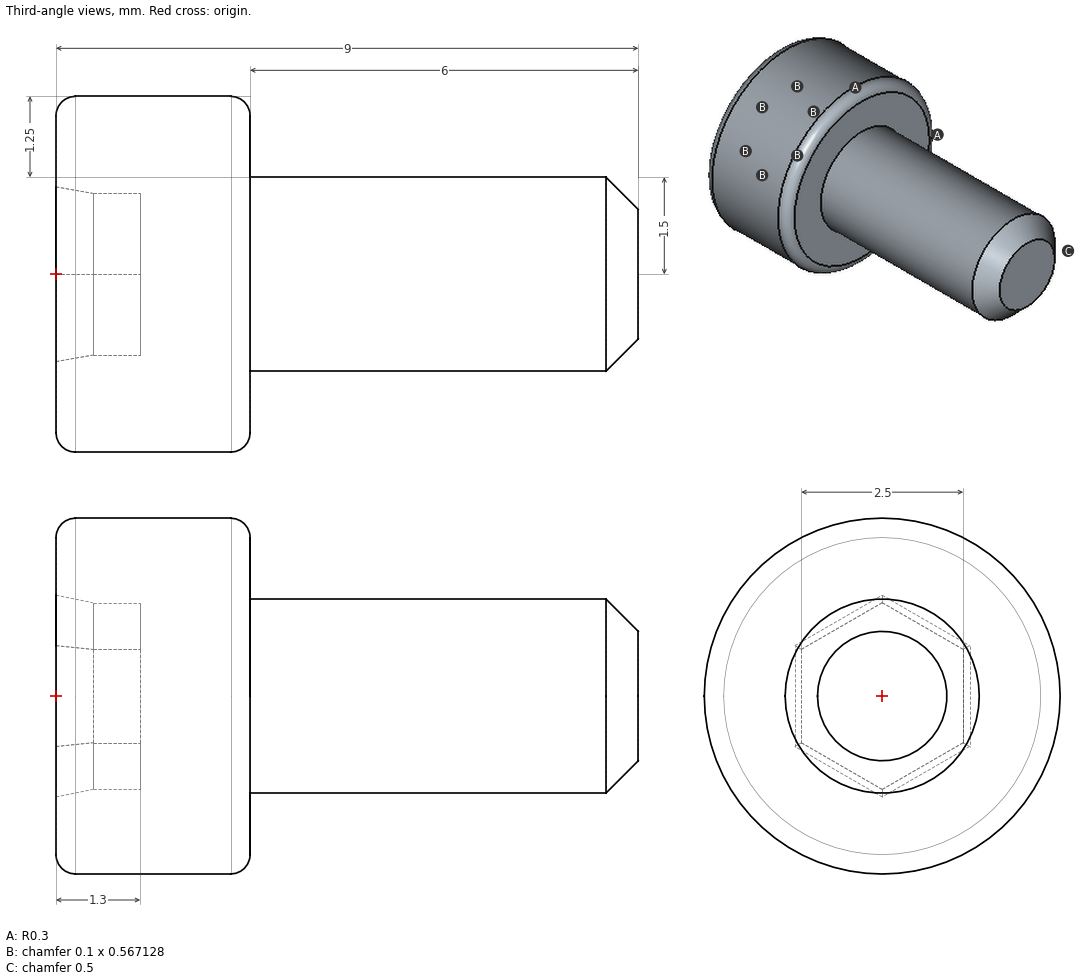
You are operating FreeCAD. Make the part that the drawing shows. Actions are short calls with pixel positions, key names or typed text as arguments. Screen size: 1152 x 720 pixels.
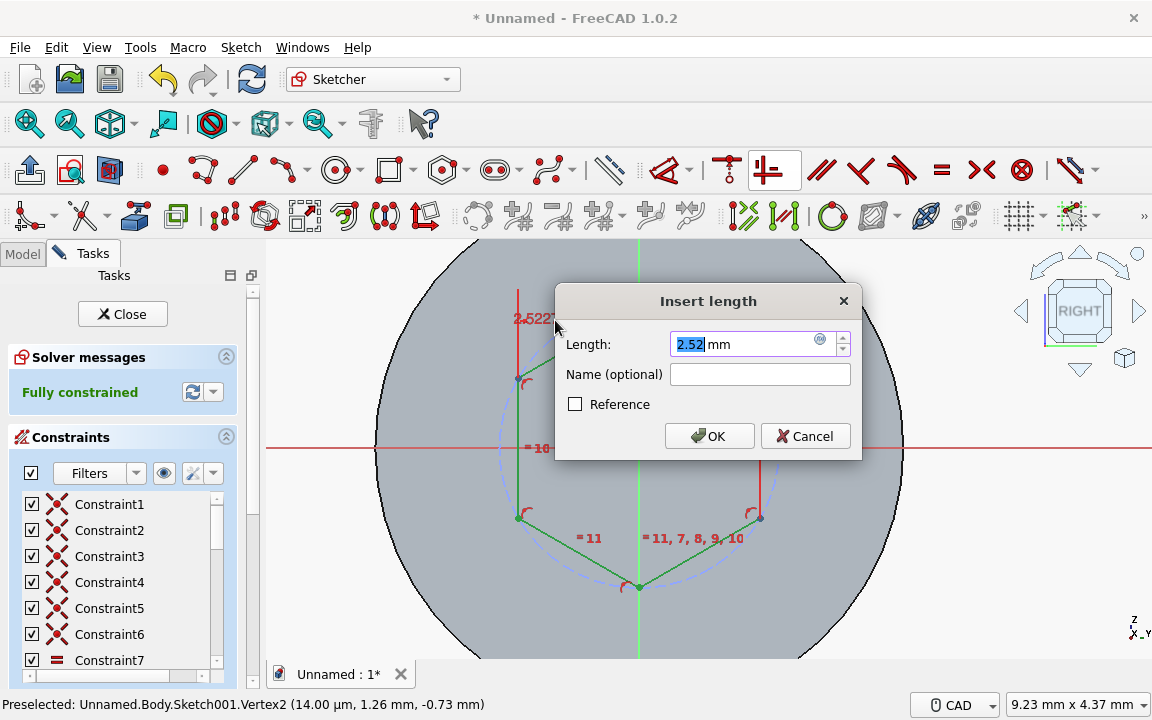
text(2.5)
key(Return)
key(Escape)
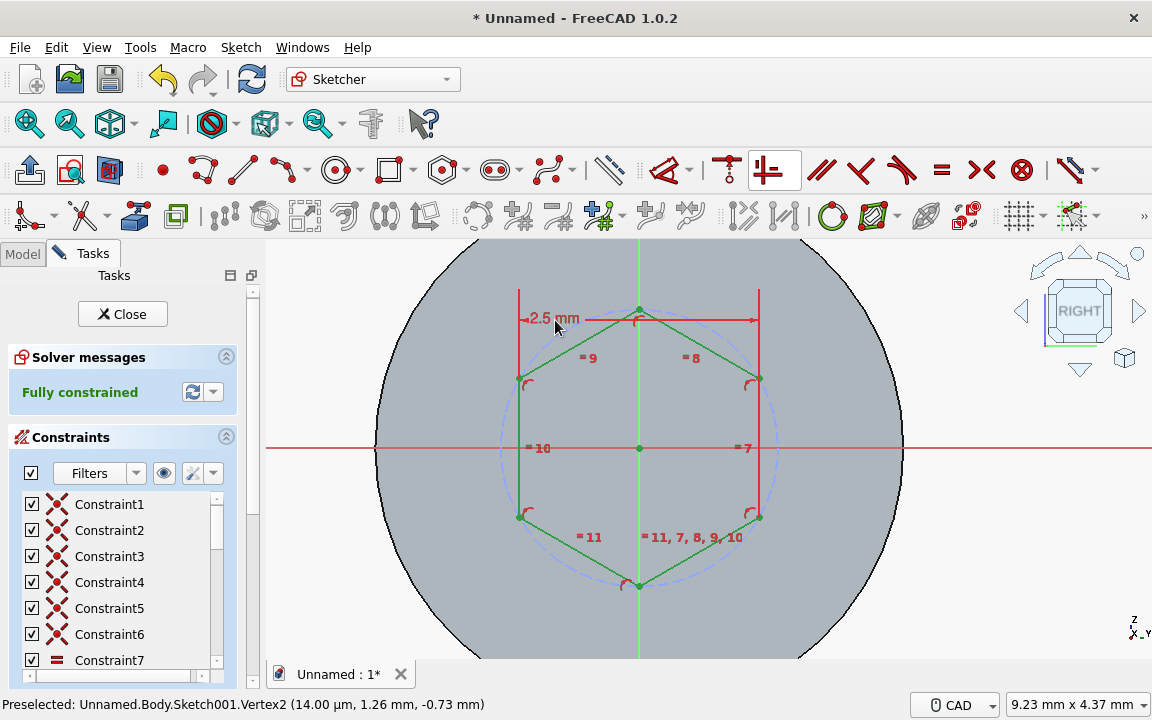
click(123, 314)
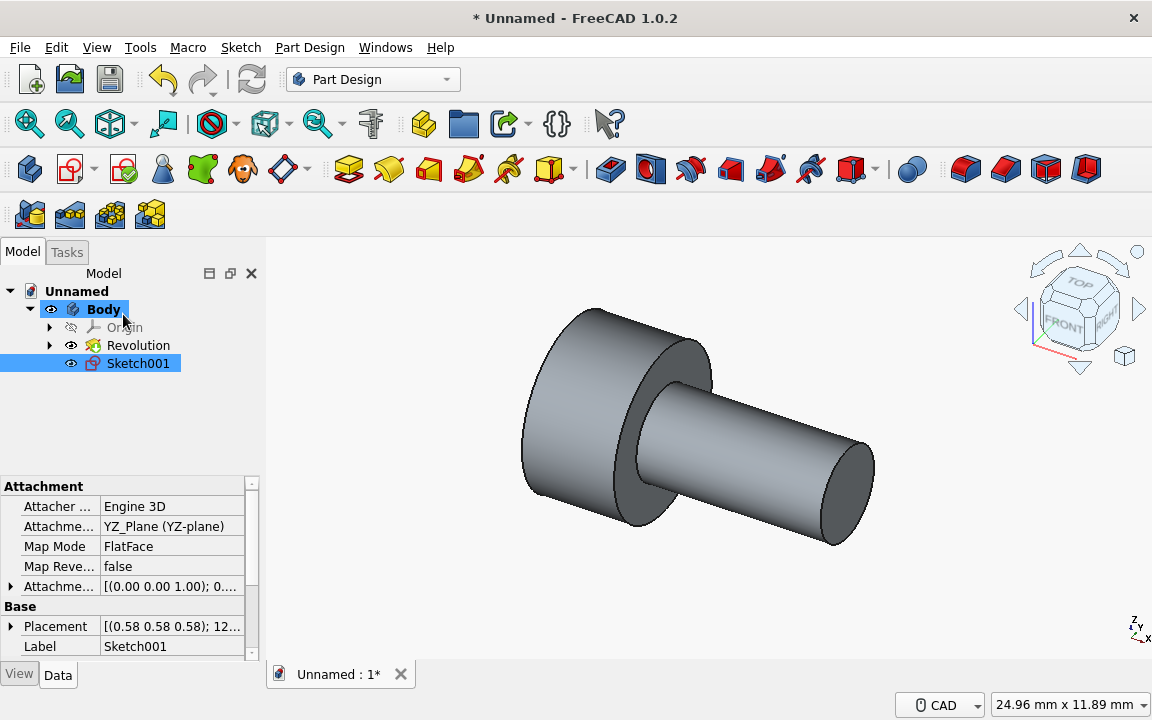
click(612, 170)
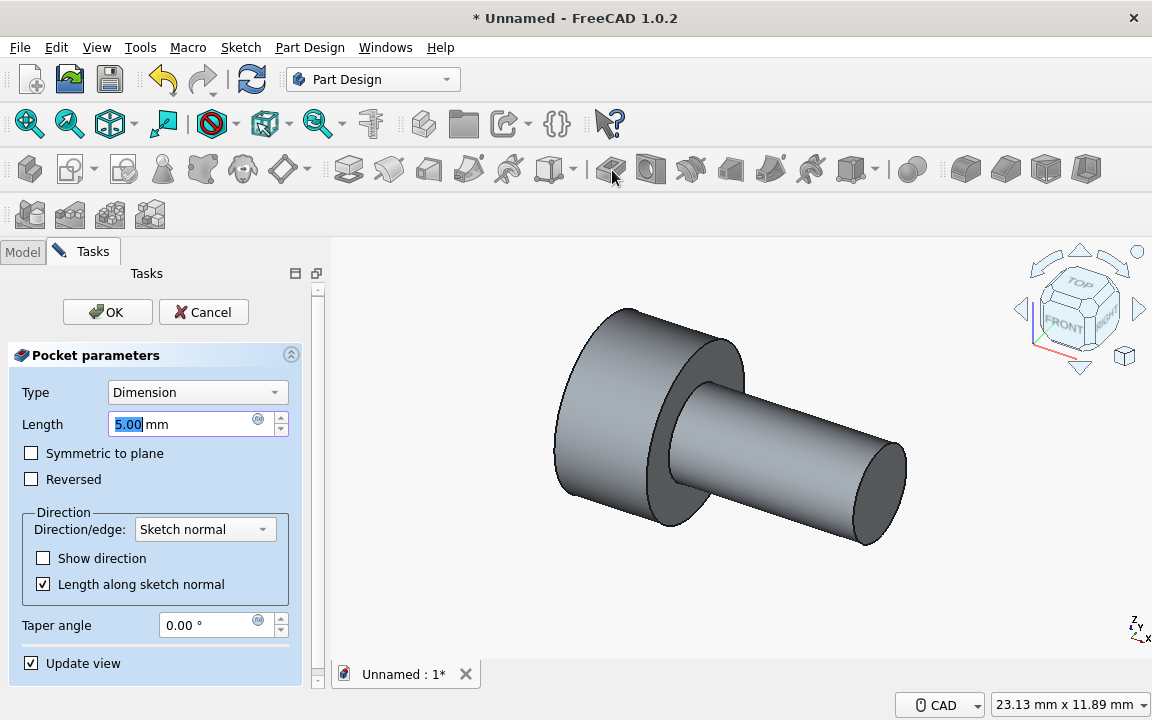
text(1.3)
key(Tab)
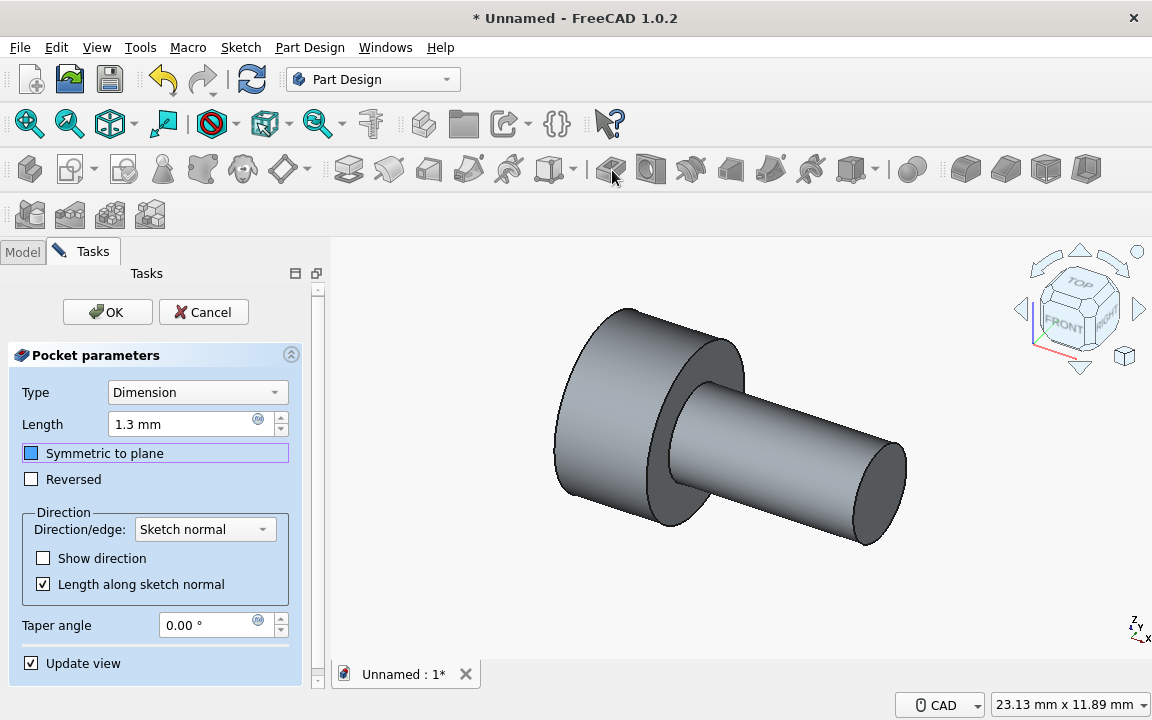
click(30, 479)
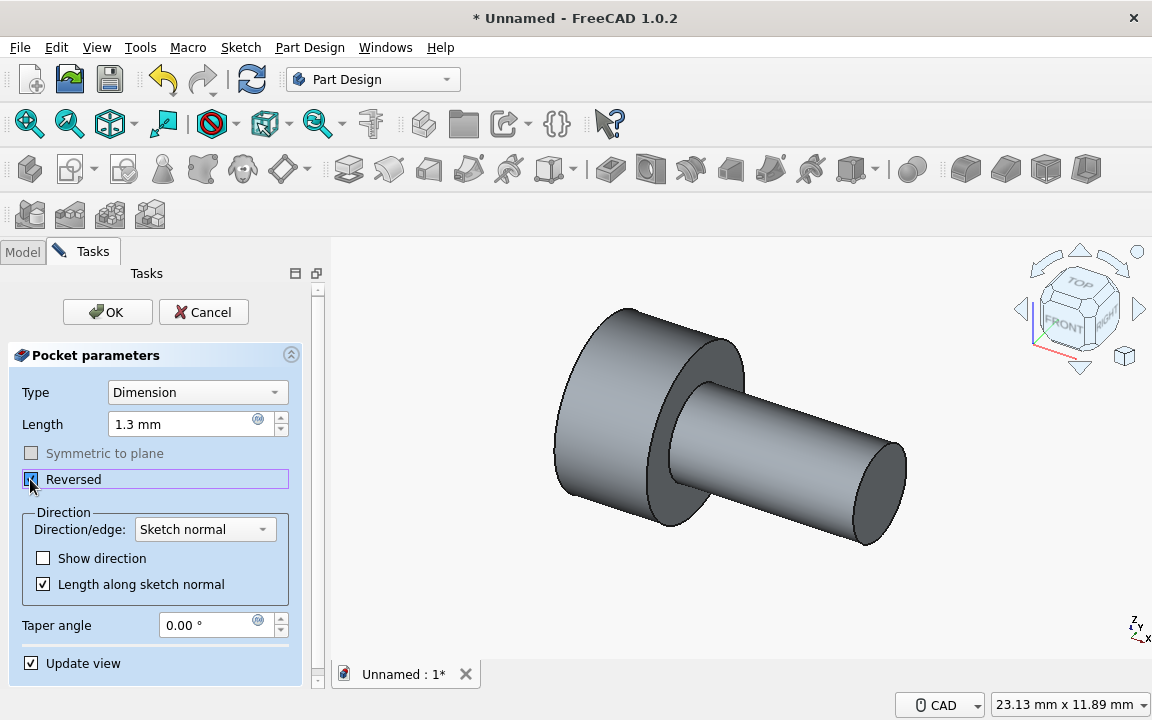
click(108, 312)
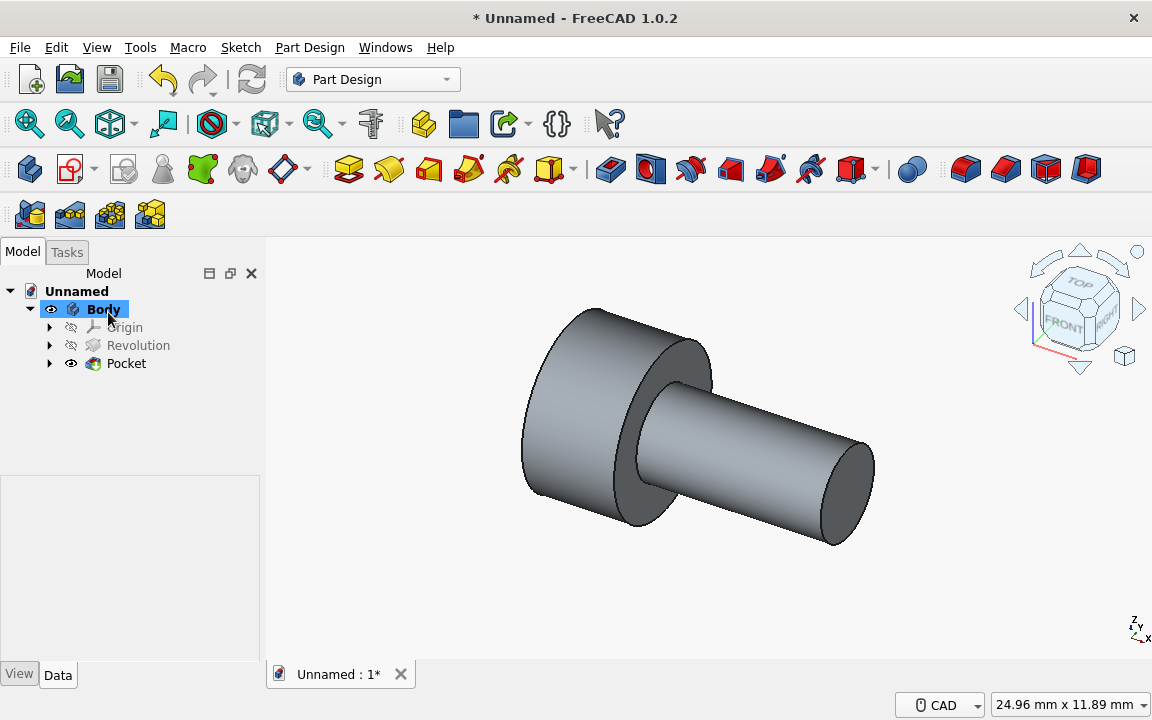
click(614, 480)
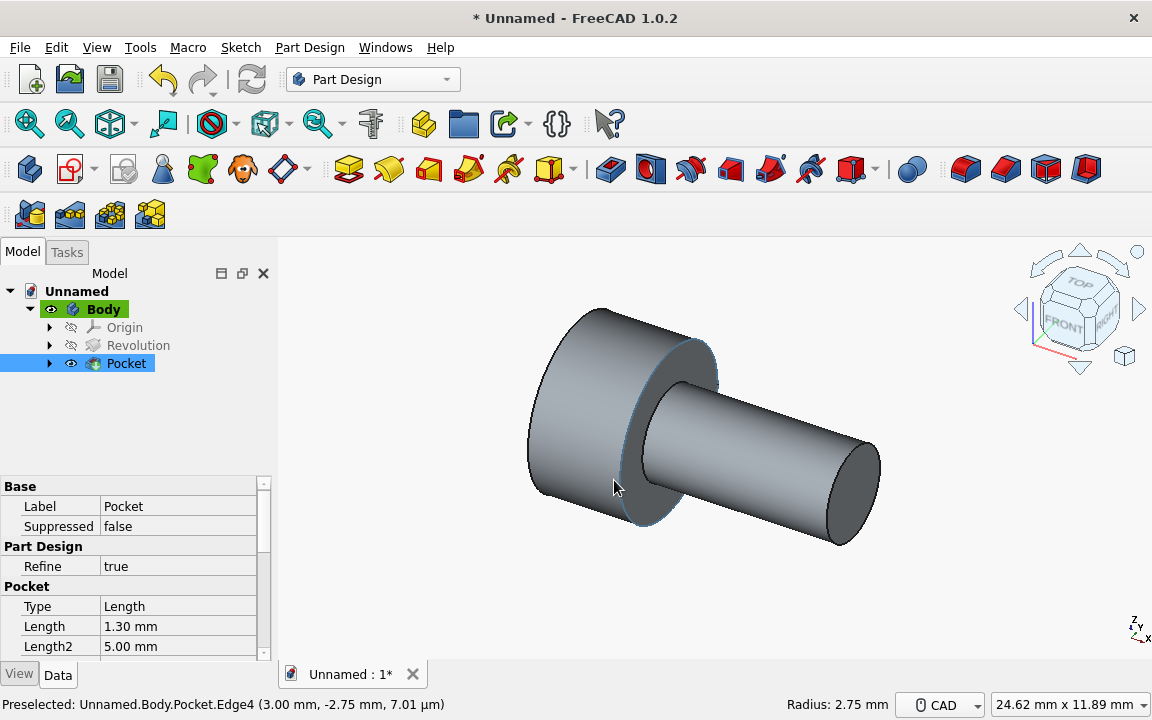
click(562, 340, ctrl)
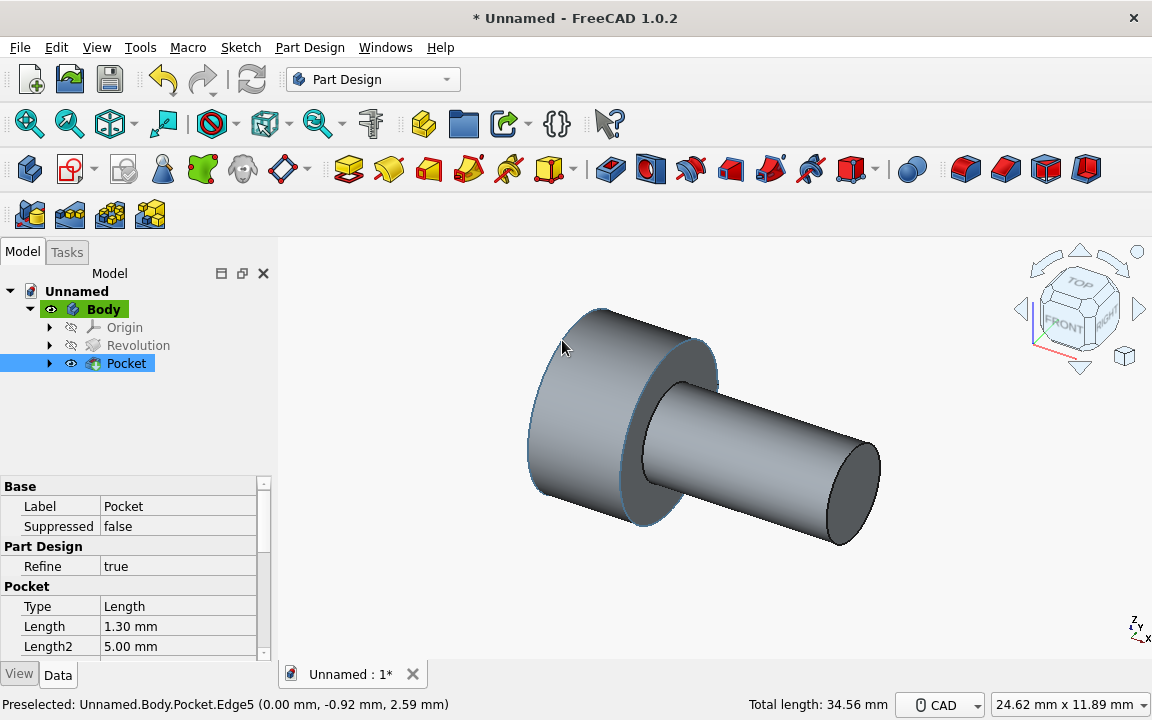
click(966, 170)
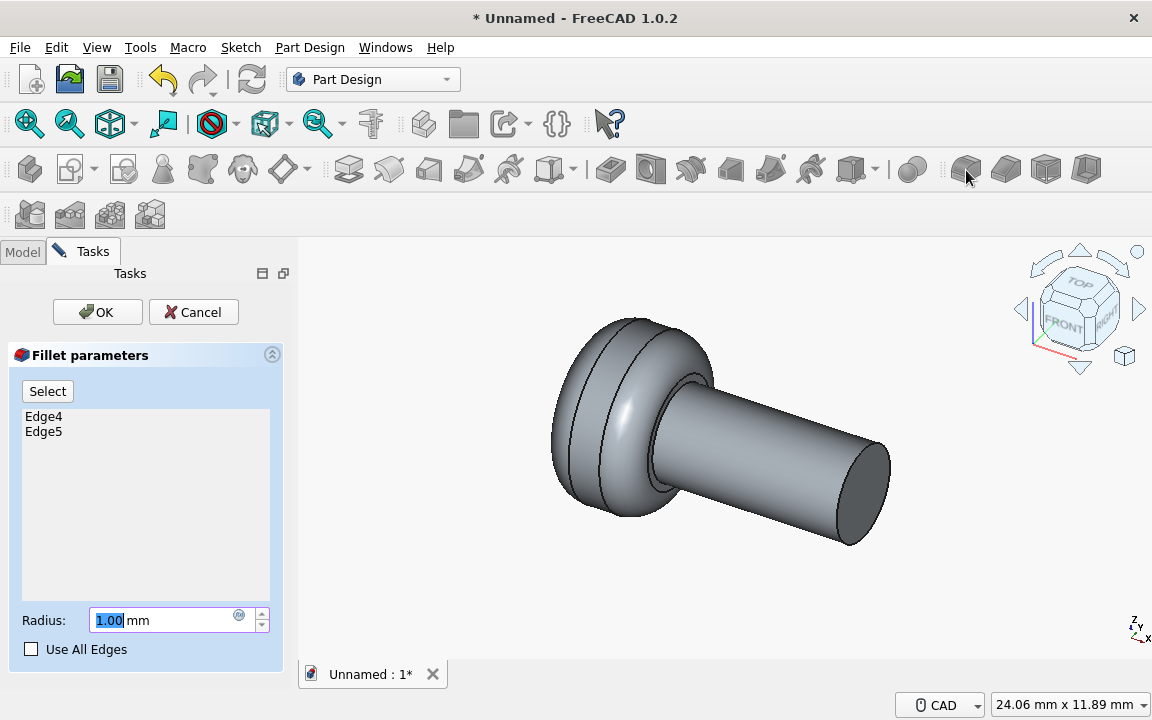
text(0.3)
key(Tab)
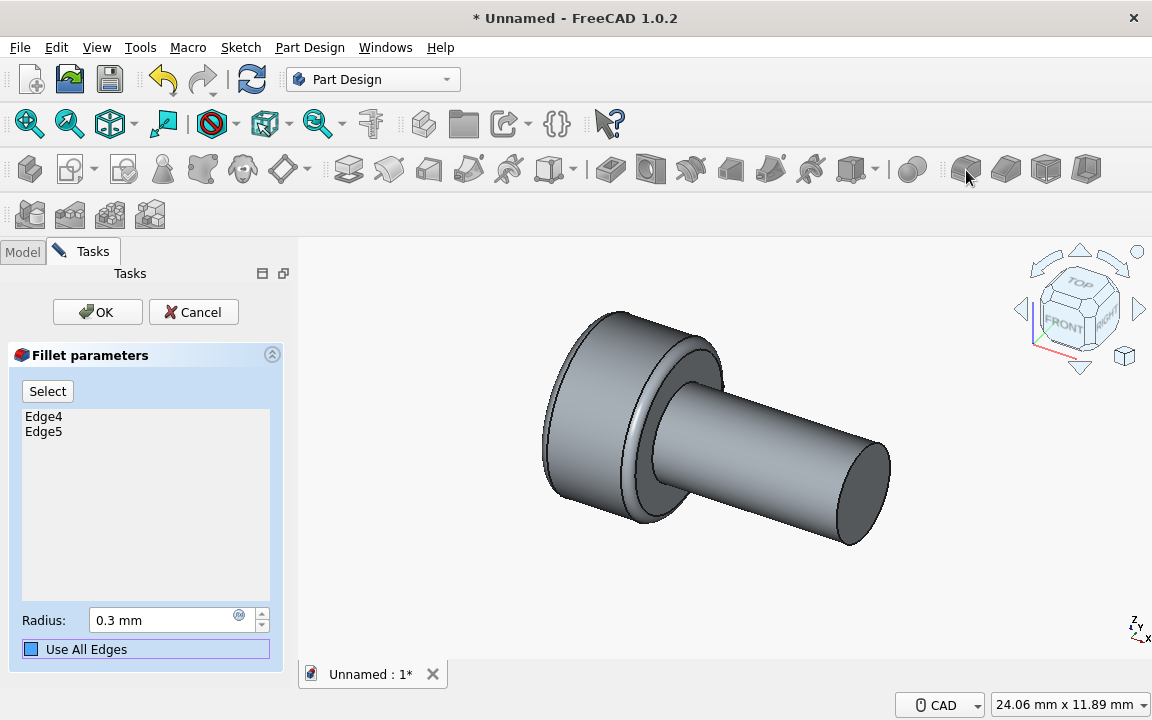
click(98, 312)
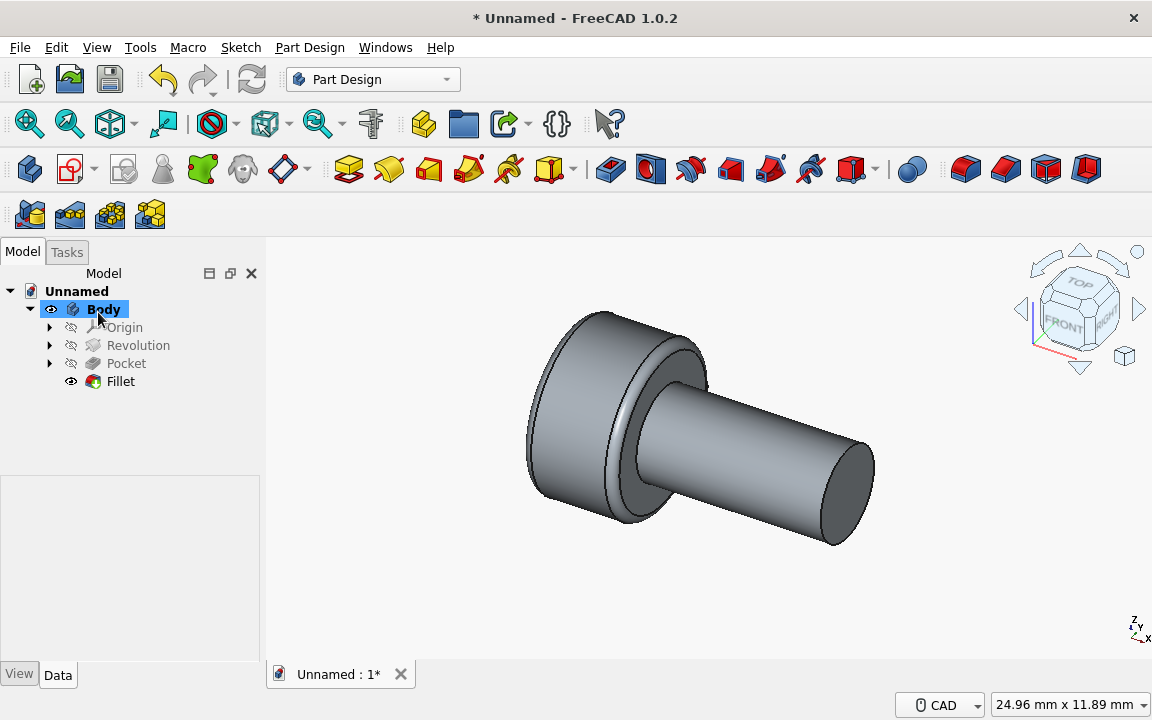
key(0)